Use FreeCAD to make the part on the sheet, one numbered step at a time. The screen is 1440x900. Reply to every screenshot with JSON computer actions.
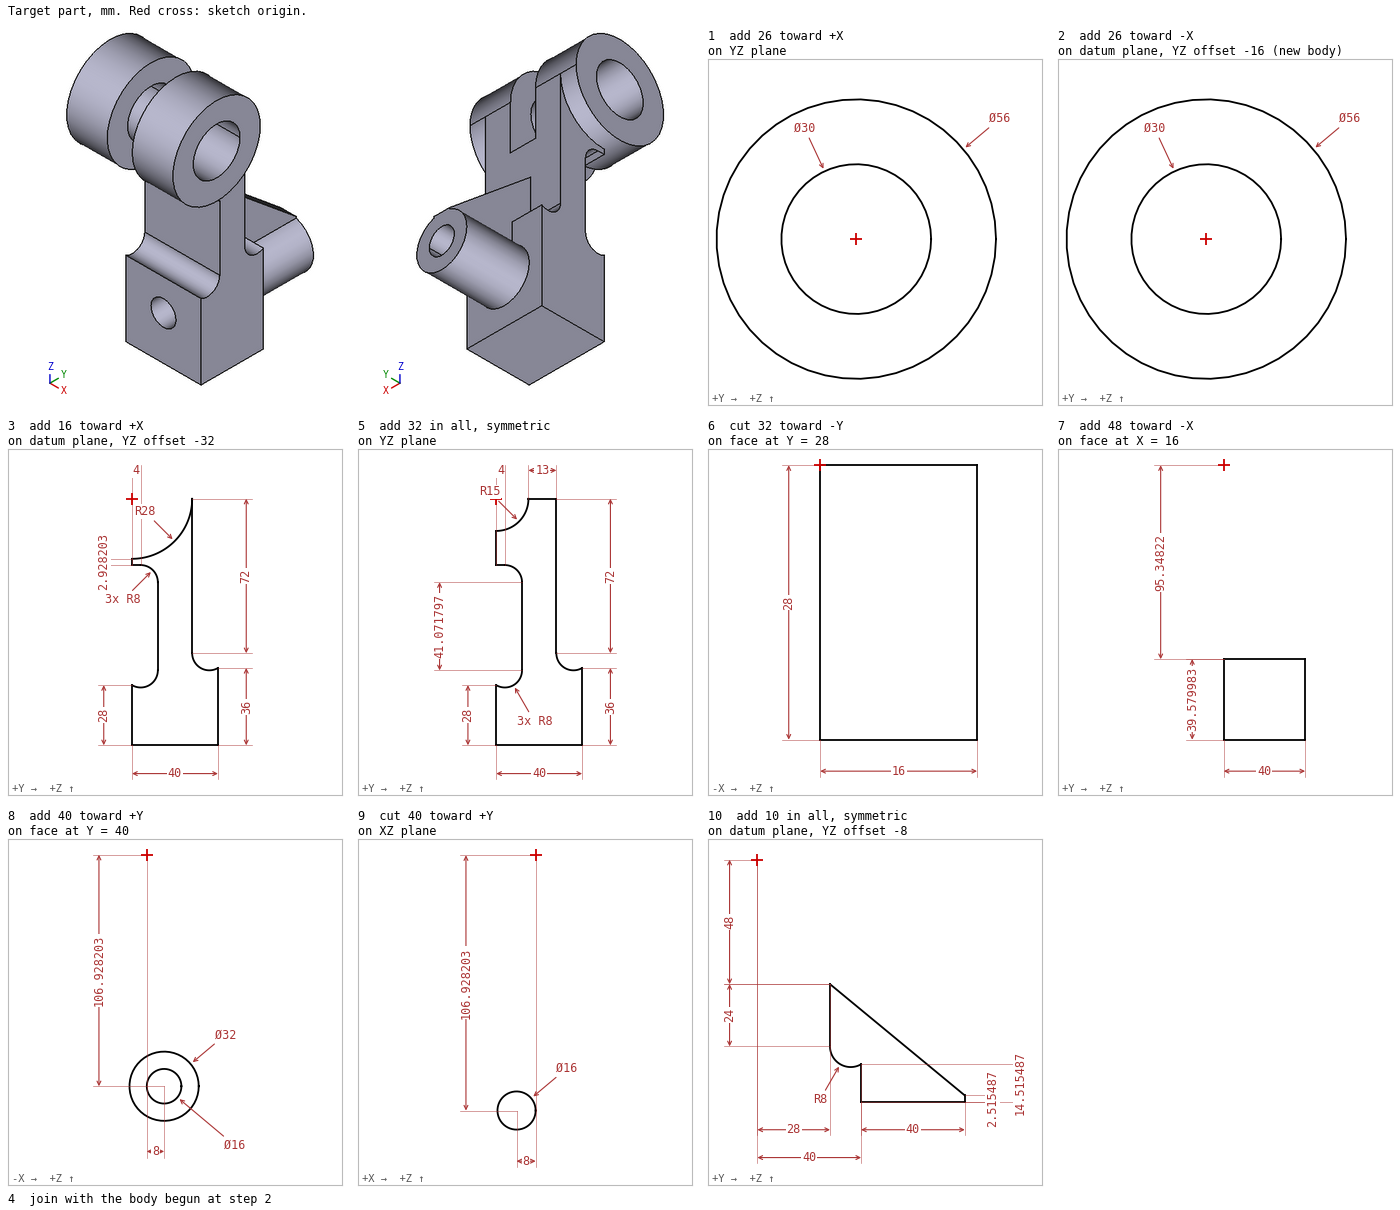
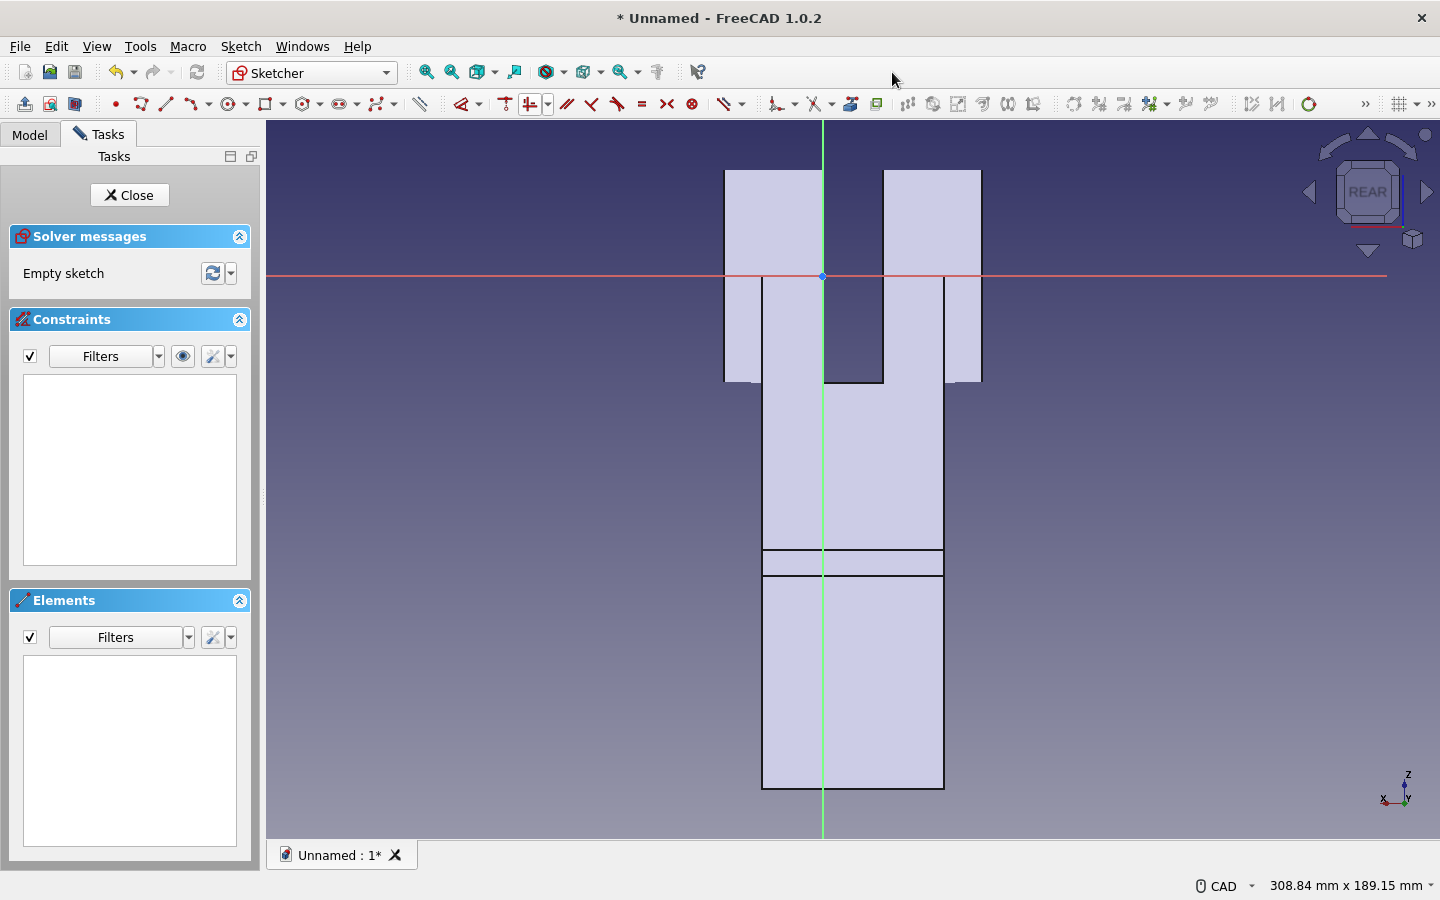
{"action": "scroll", "coordinate": [875, 749], "scroll_direction": "up", "scroll_amount": 7}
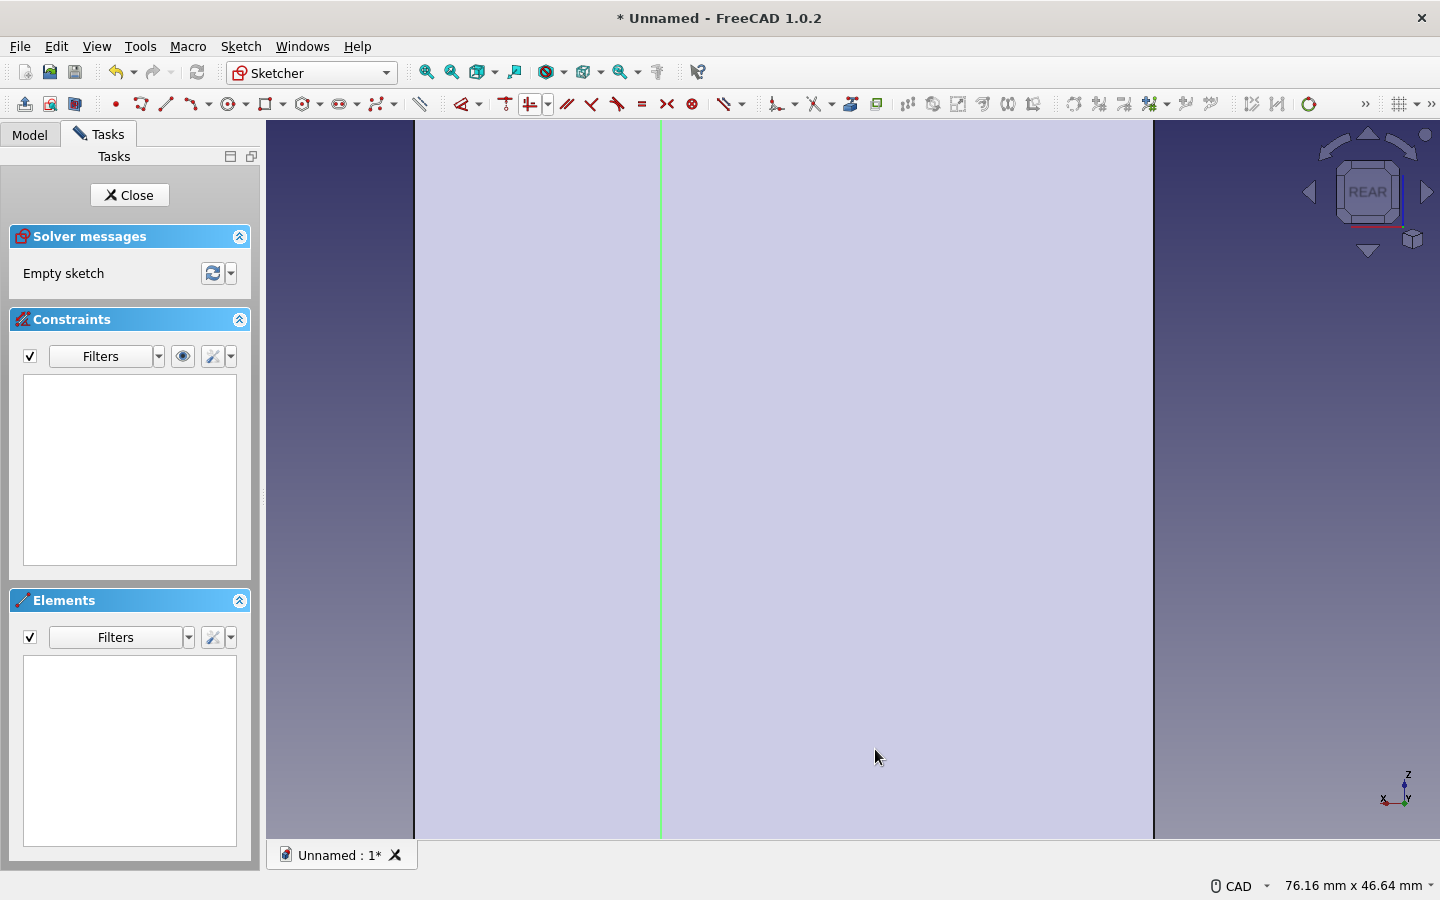
{"action": "left_click", "coordinate": [228, 104]}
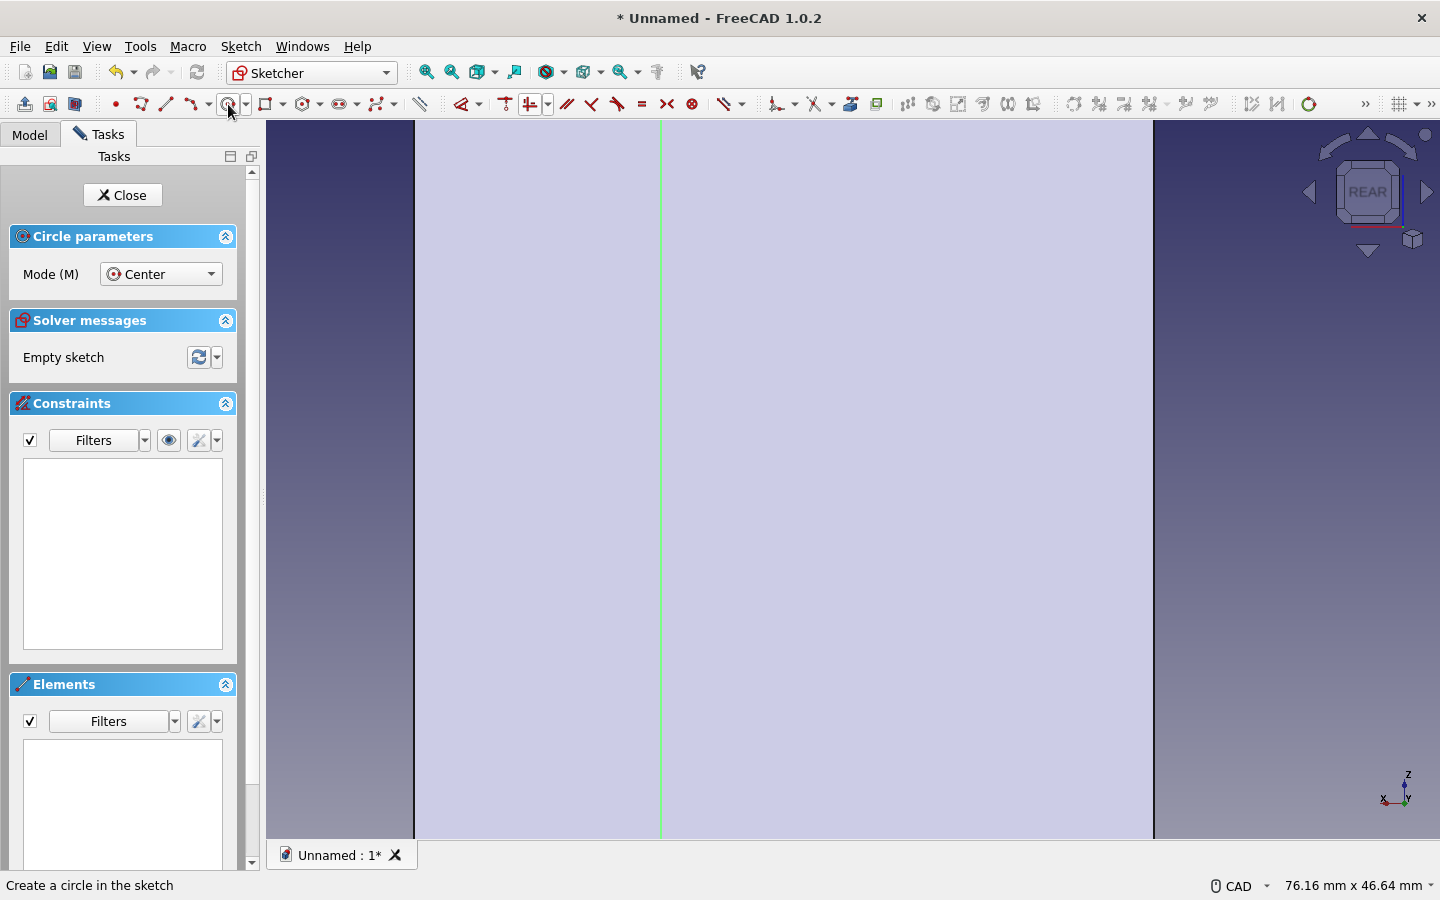
{"action": "left_click", "coordinate": [784, 477]}
{"action": "left_click", "coordinate": [959, 303]}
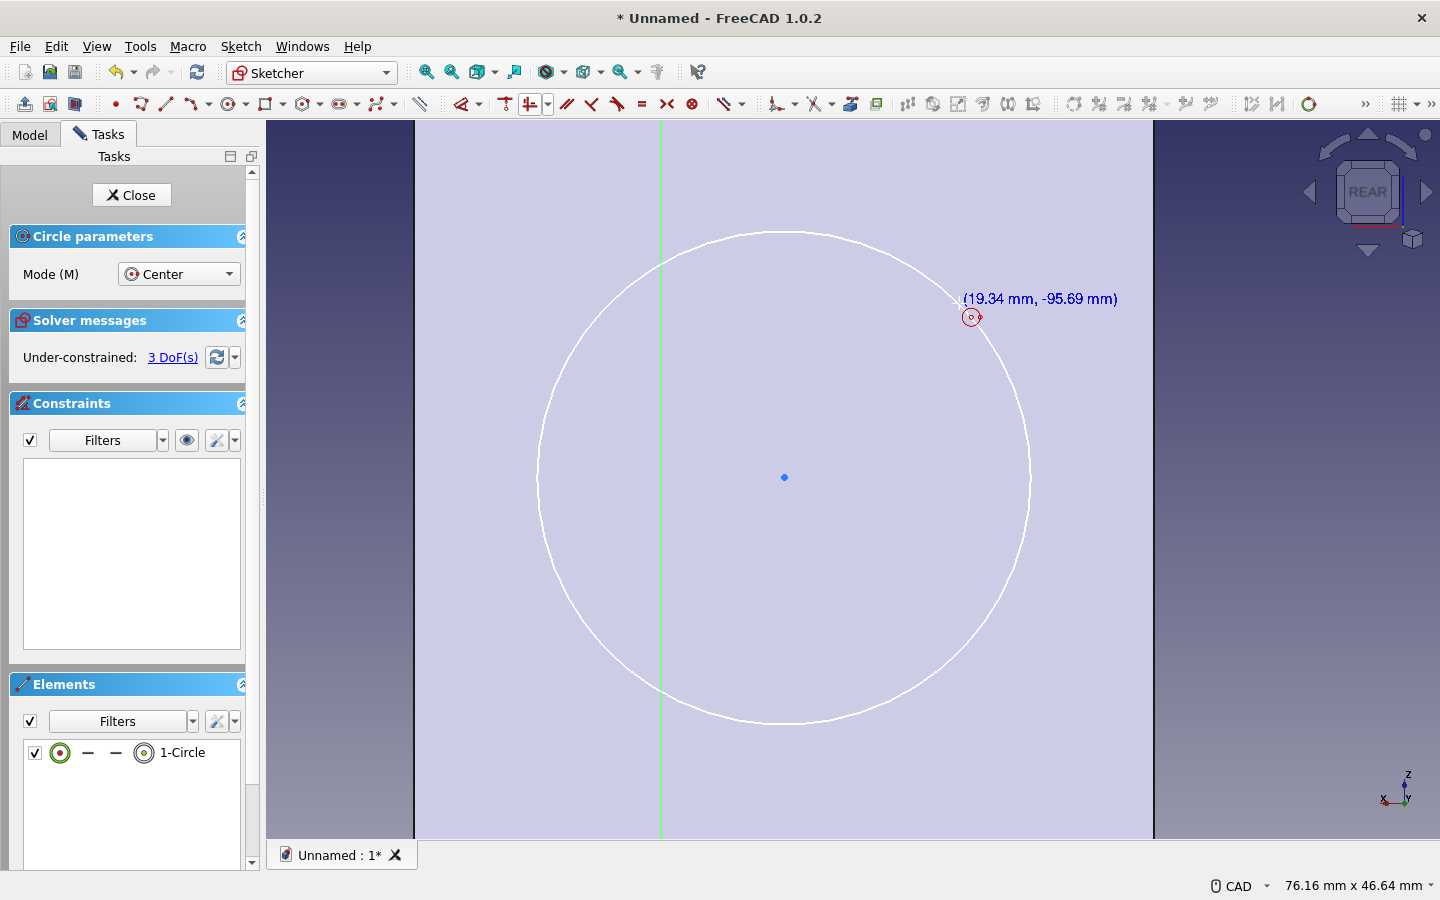
{"action": "left_click", "coordinate": [784, 478]}
{"action": "left_click", "coordinate": [871, 390]}
{"action": "key", "text": "Escape"}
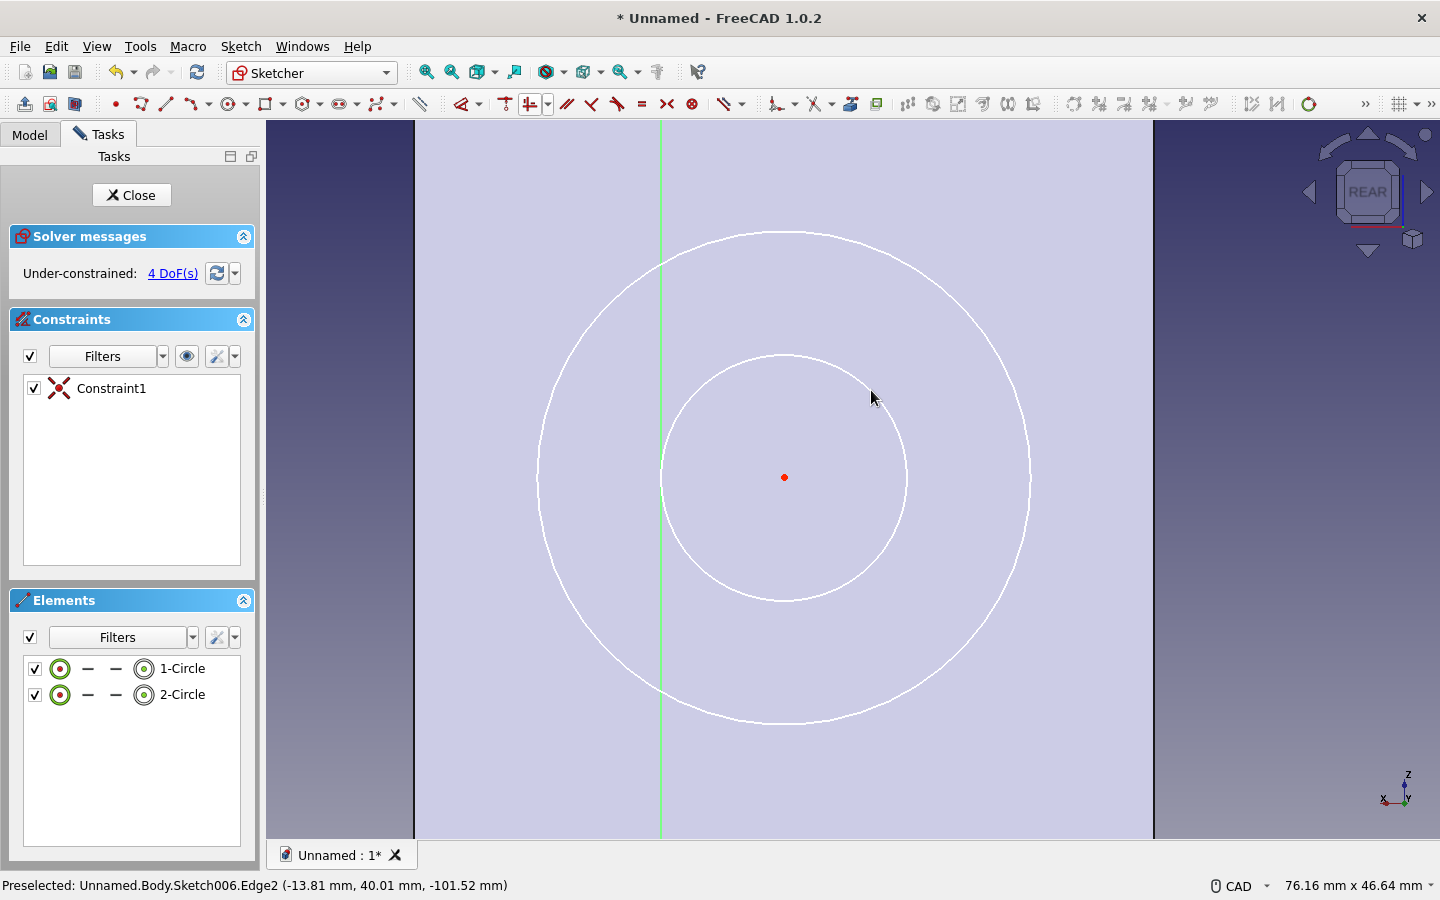
{"action": "key", "text": "d"}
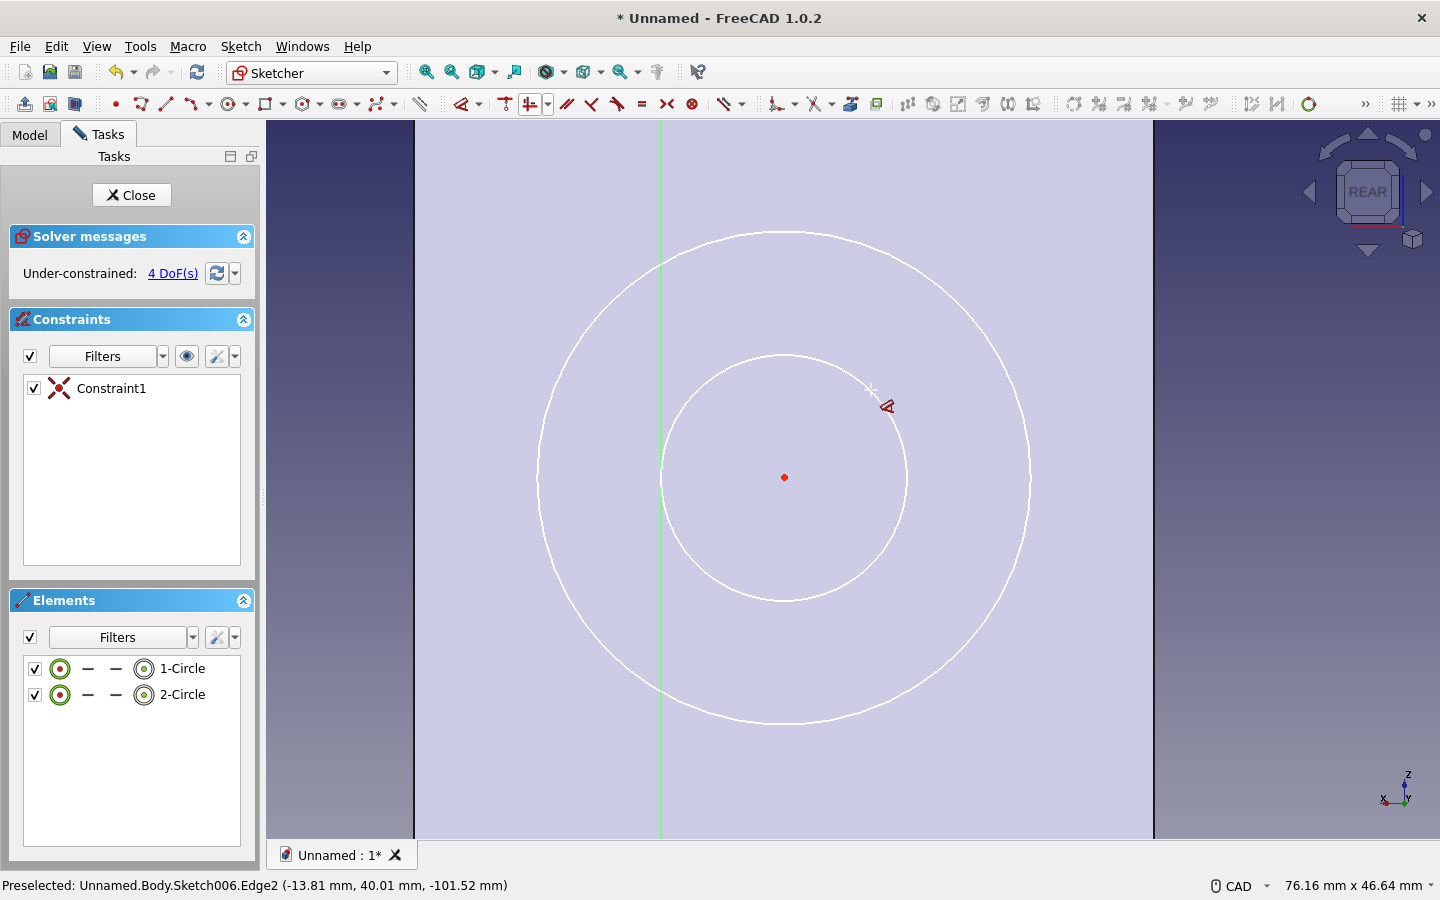
{"action": "left_click", "coordinate": [958, 303]}
{"action": "left_click", "coordinate": [981, 280]}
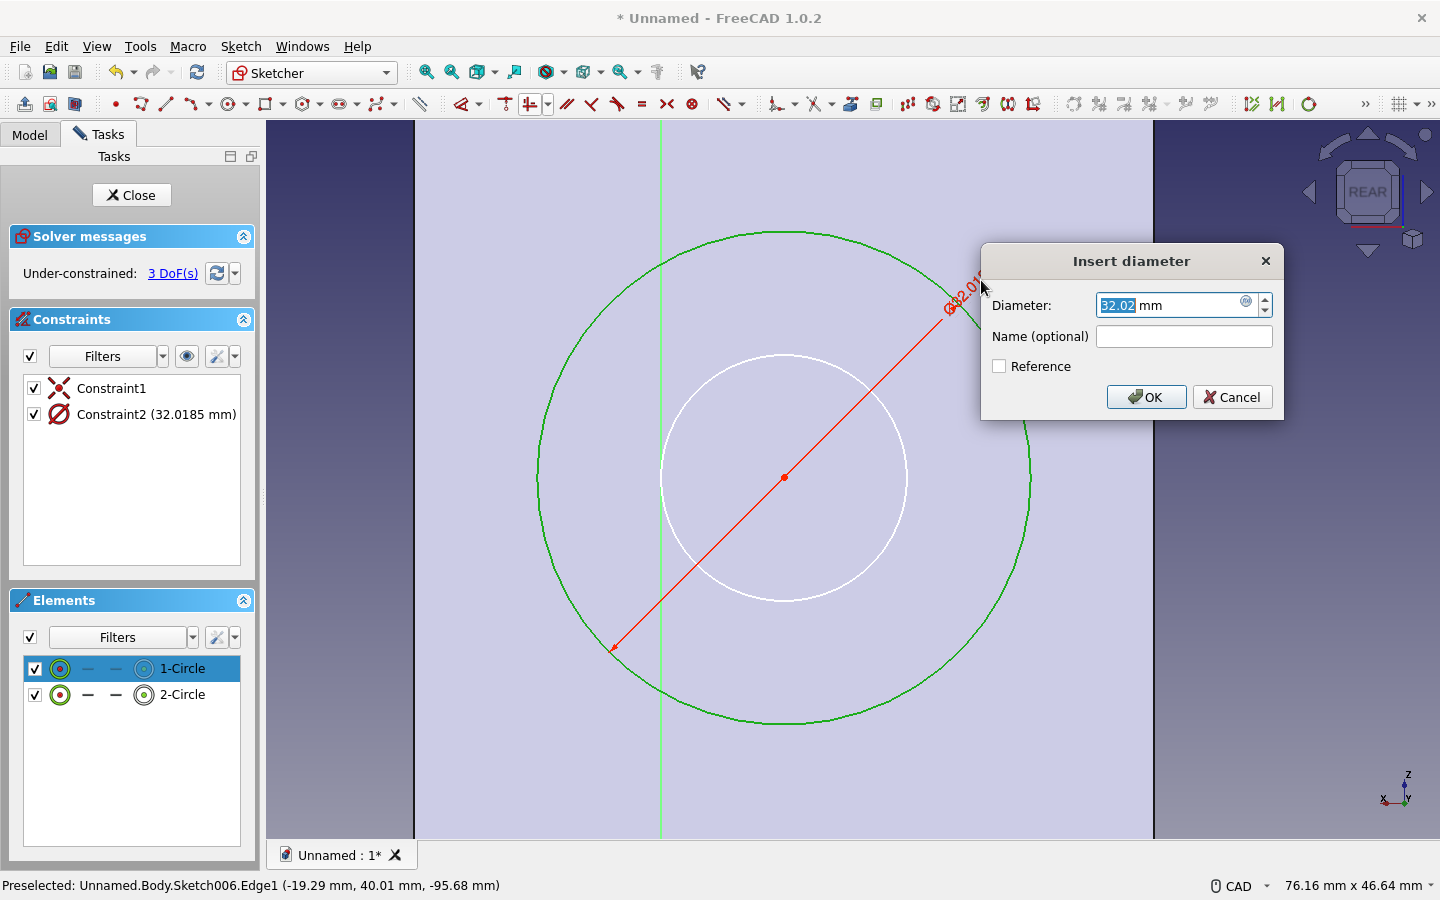
{"action": "type", "text": "32"}
{"action": "key", "text": "Return"}